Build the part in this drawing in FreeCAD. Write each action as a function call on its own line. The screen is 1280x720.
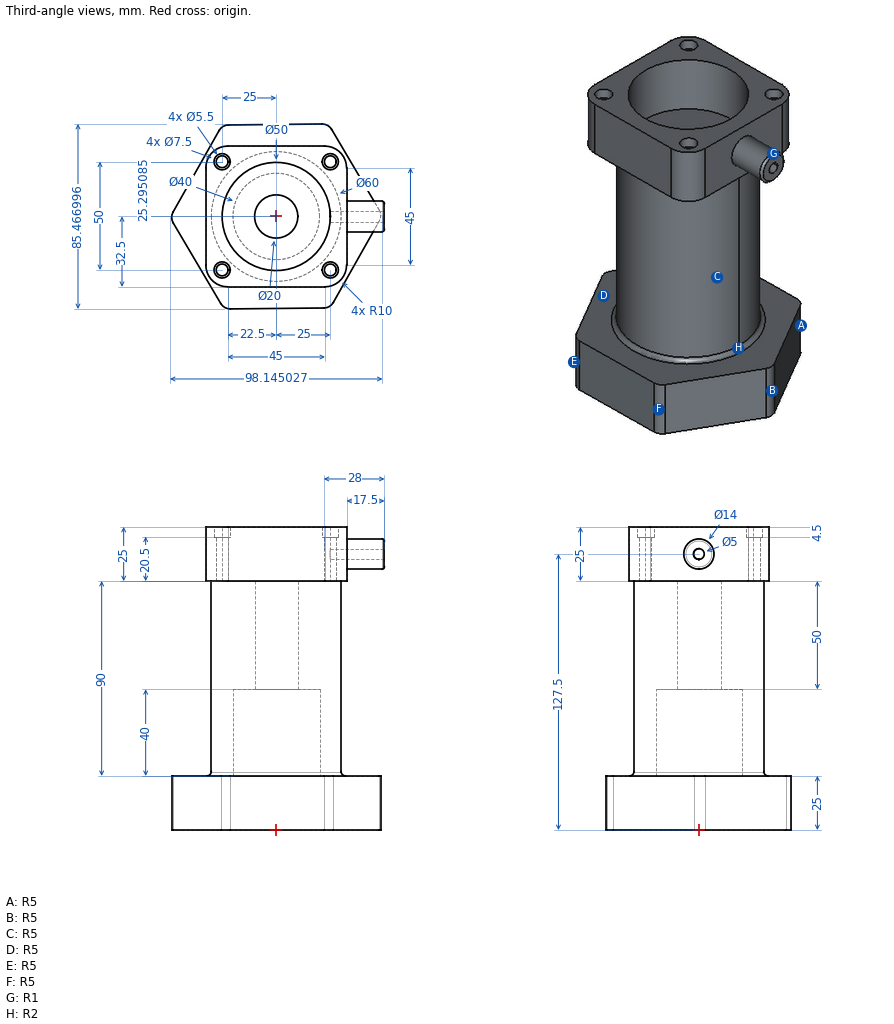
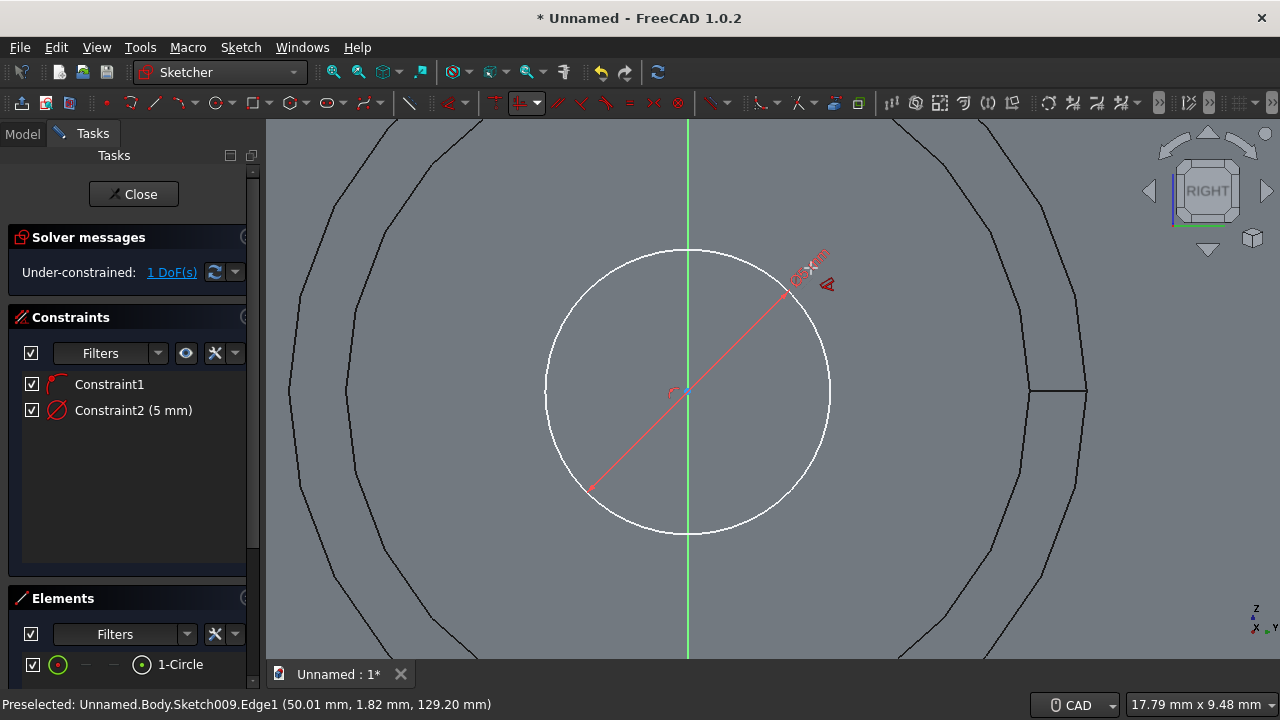
click(688, 392)
click(722, 512)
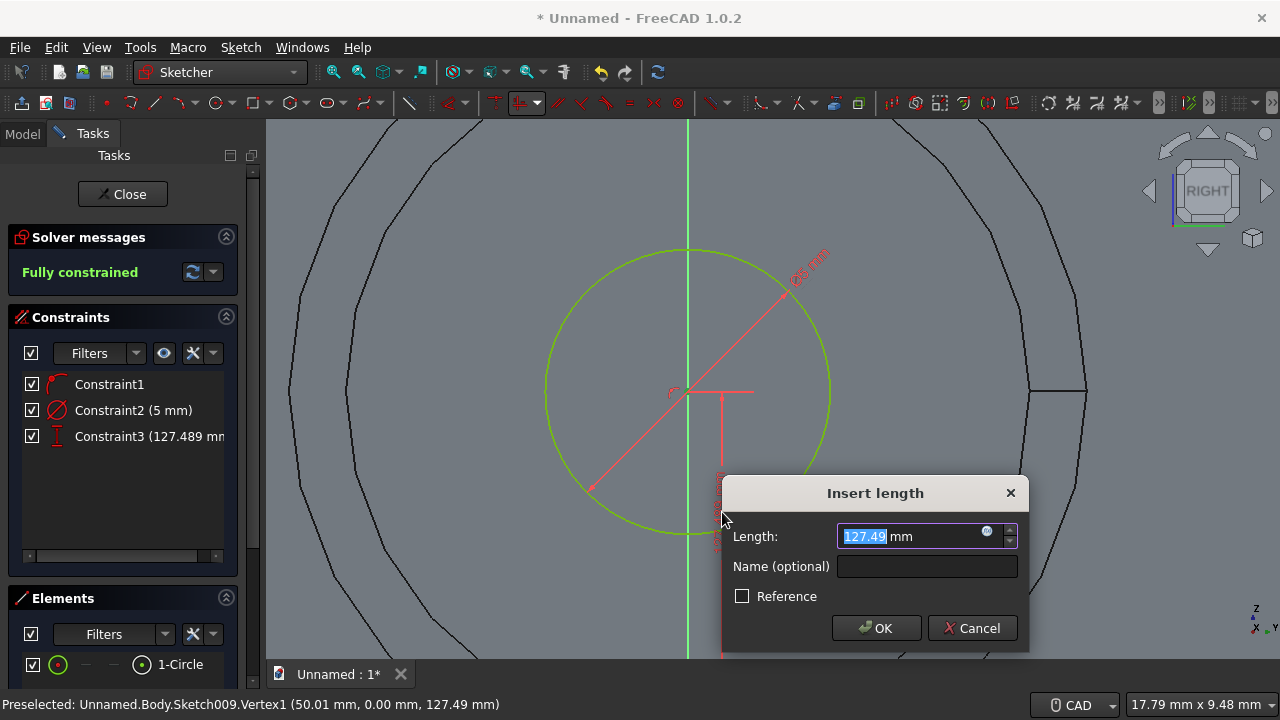
text(127.5)
key(Return)
key(Escape)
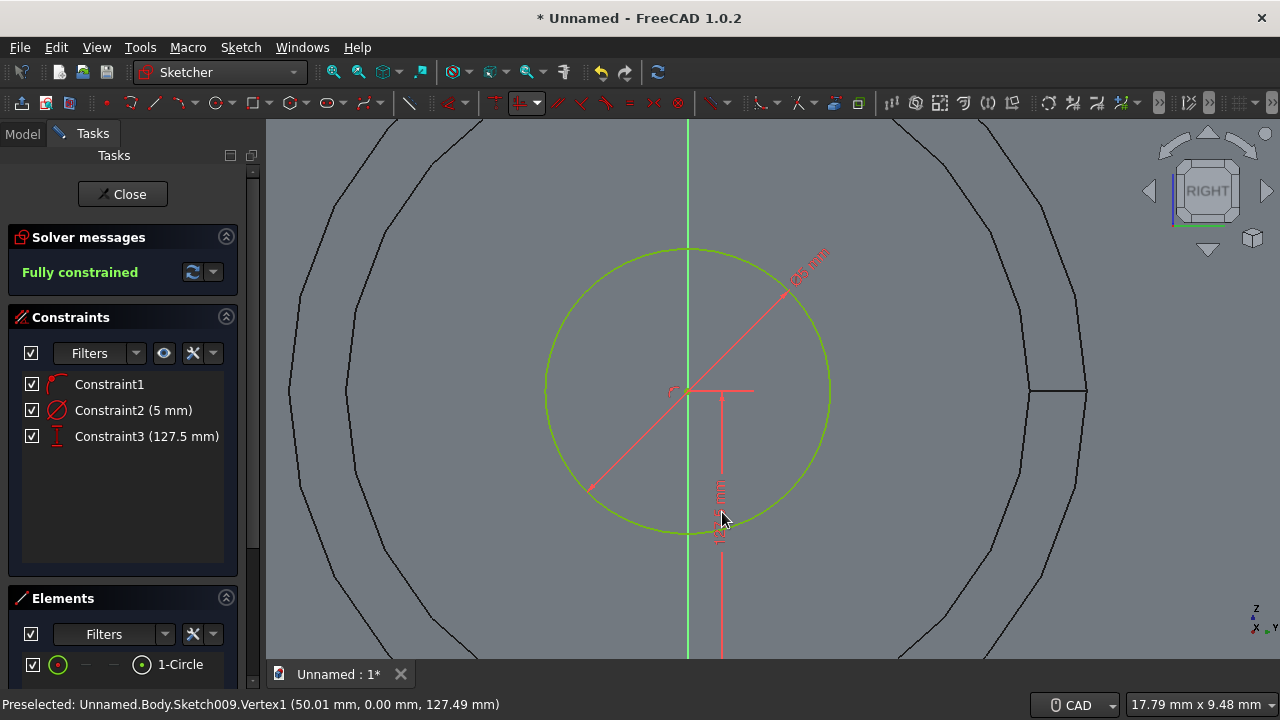
click(123, 194)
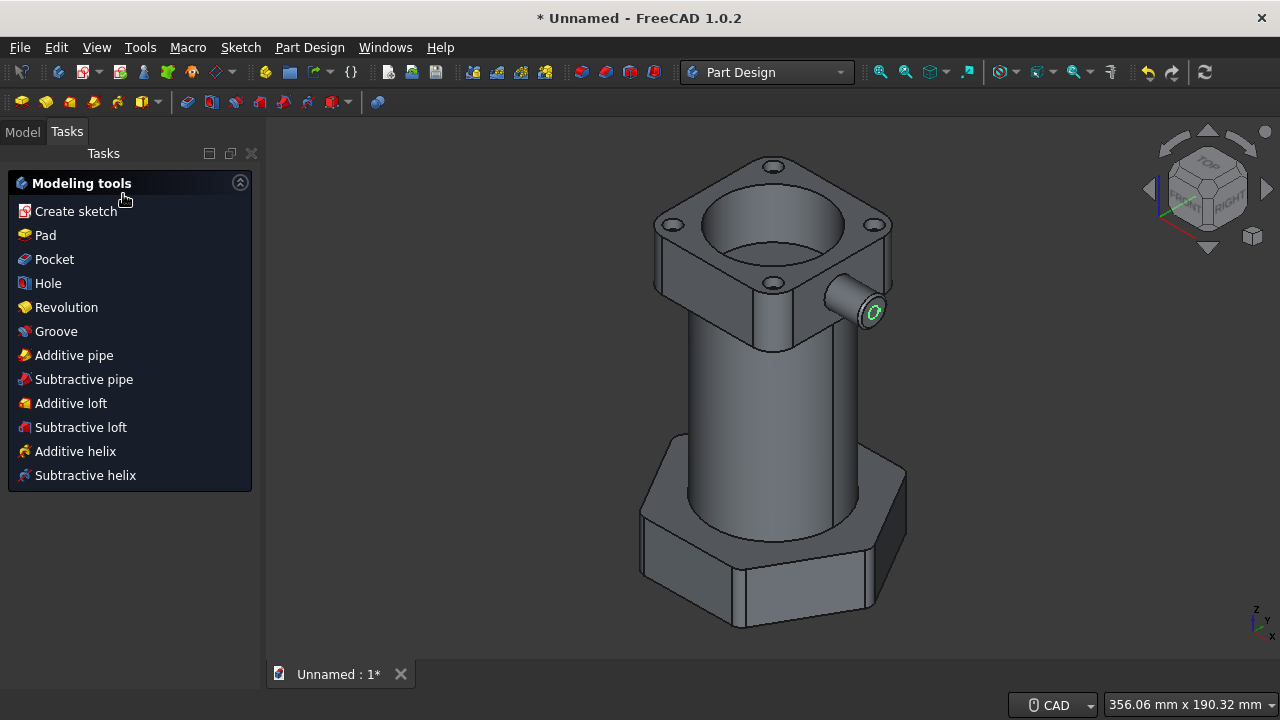
click(188, 102)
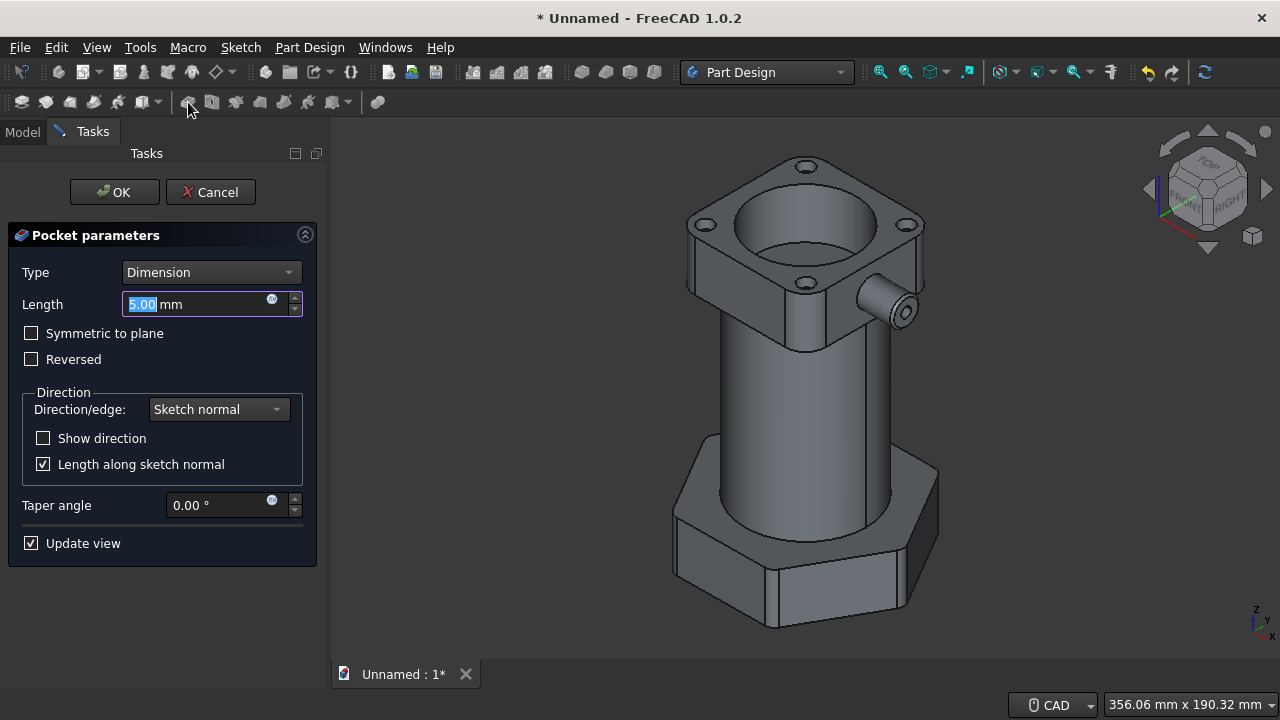
text(28)
key(Tab)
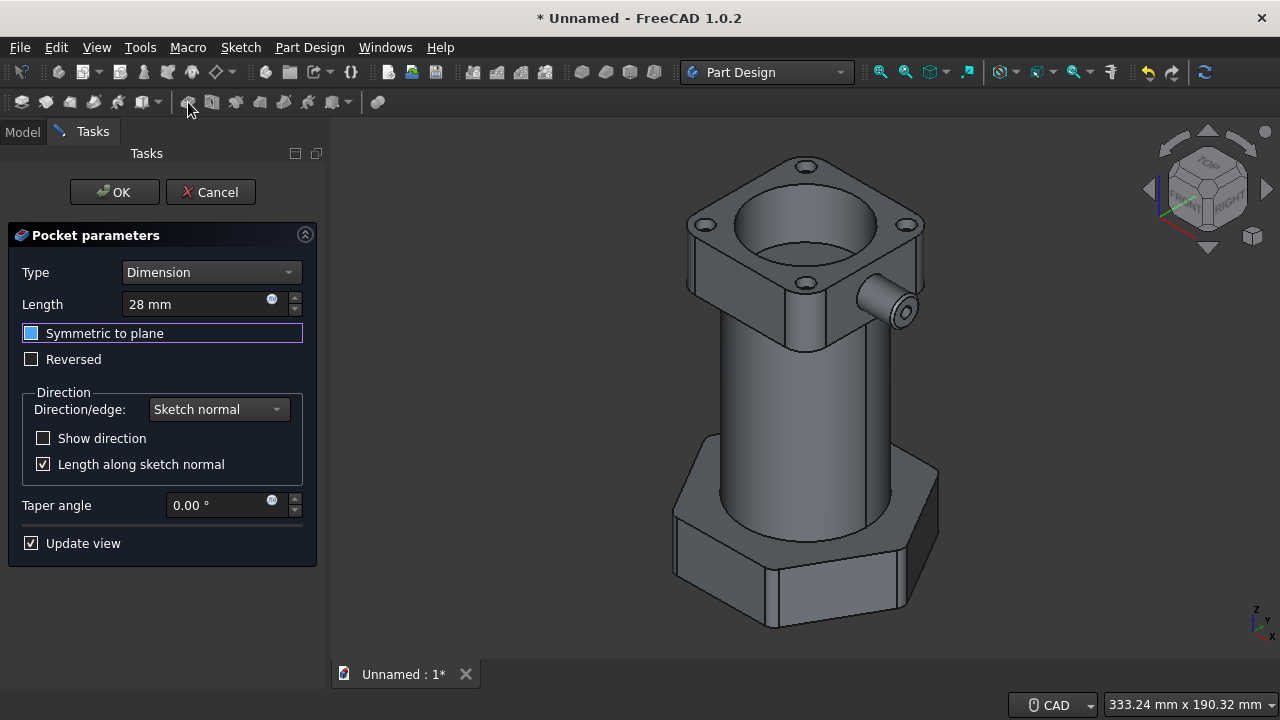
click(115, 192)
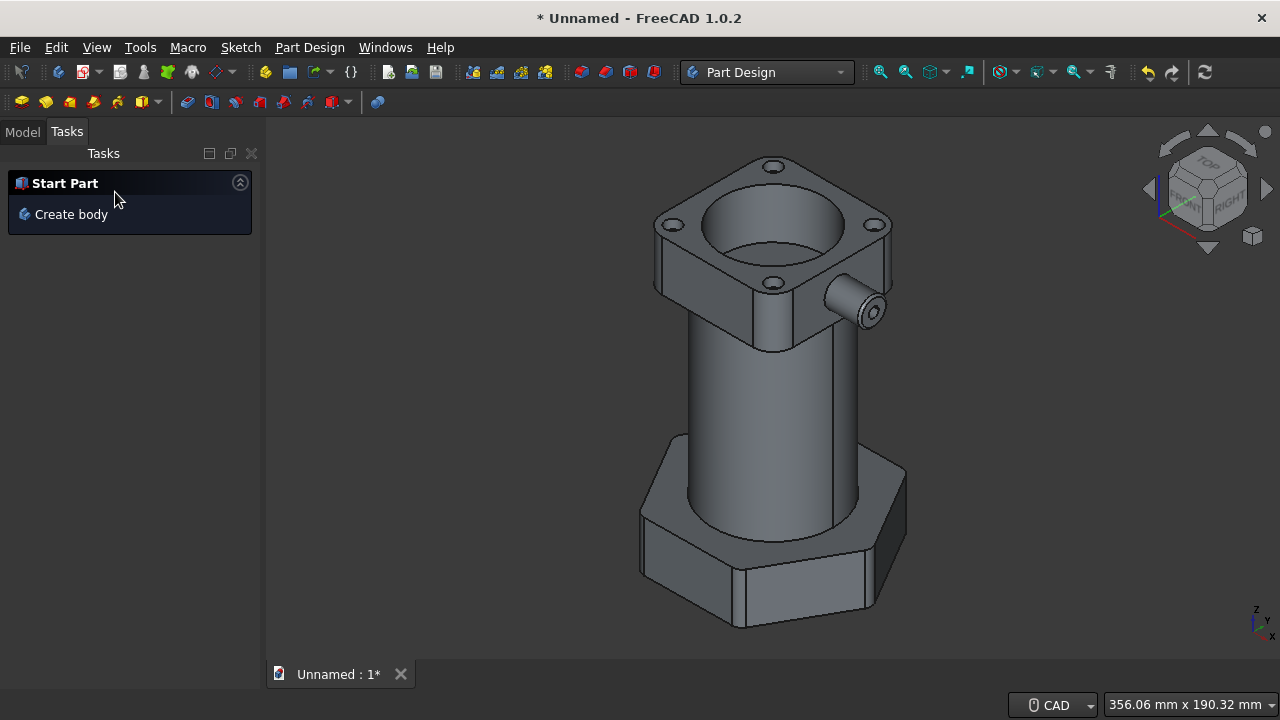
key(2)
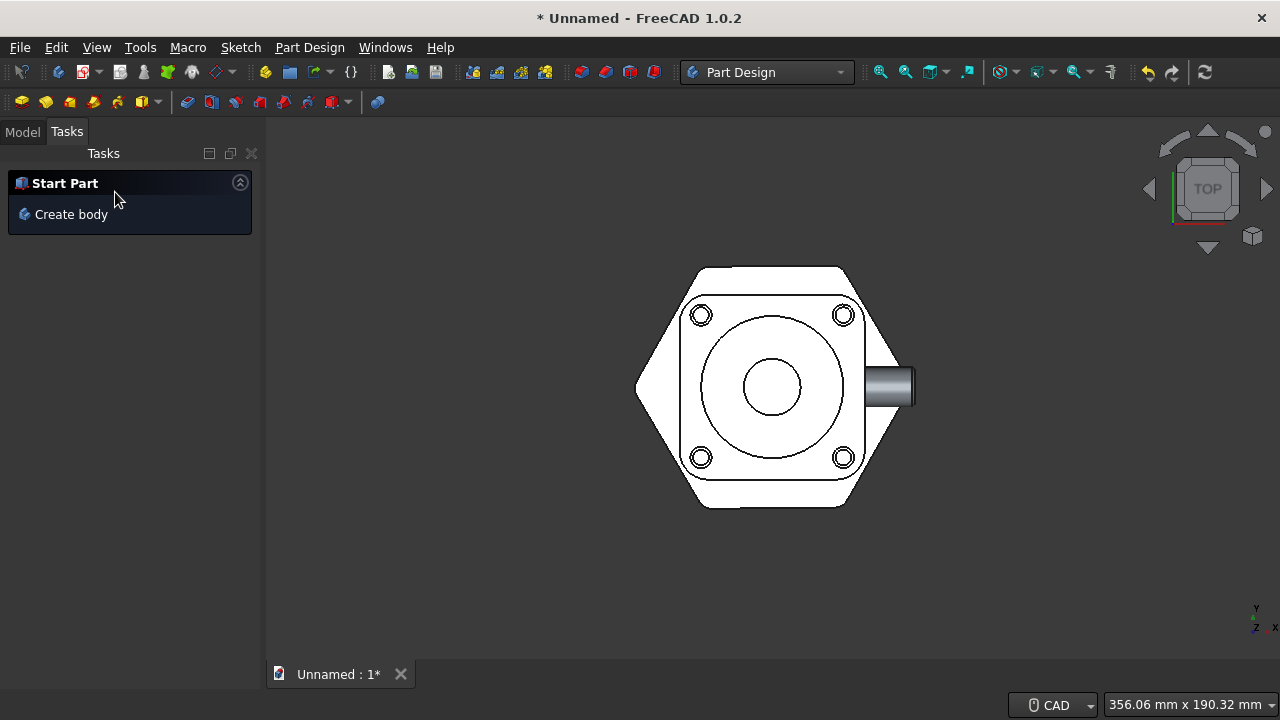
click(882, 72)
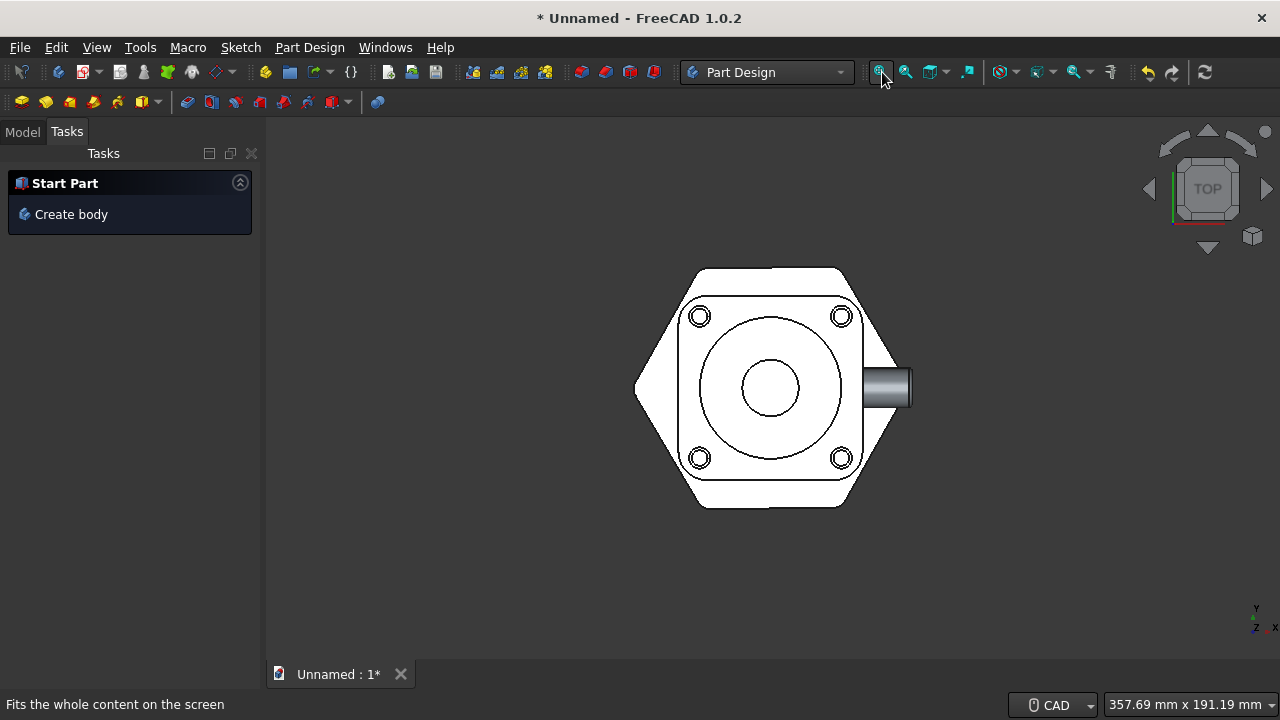
key(0)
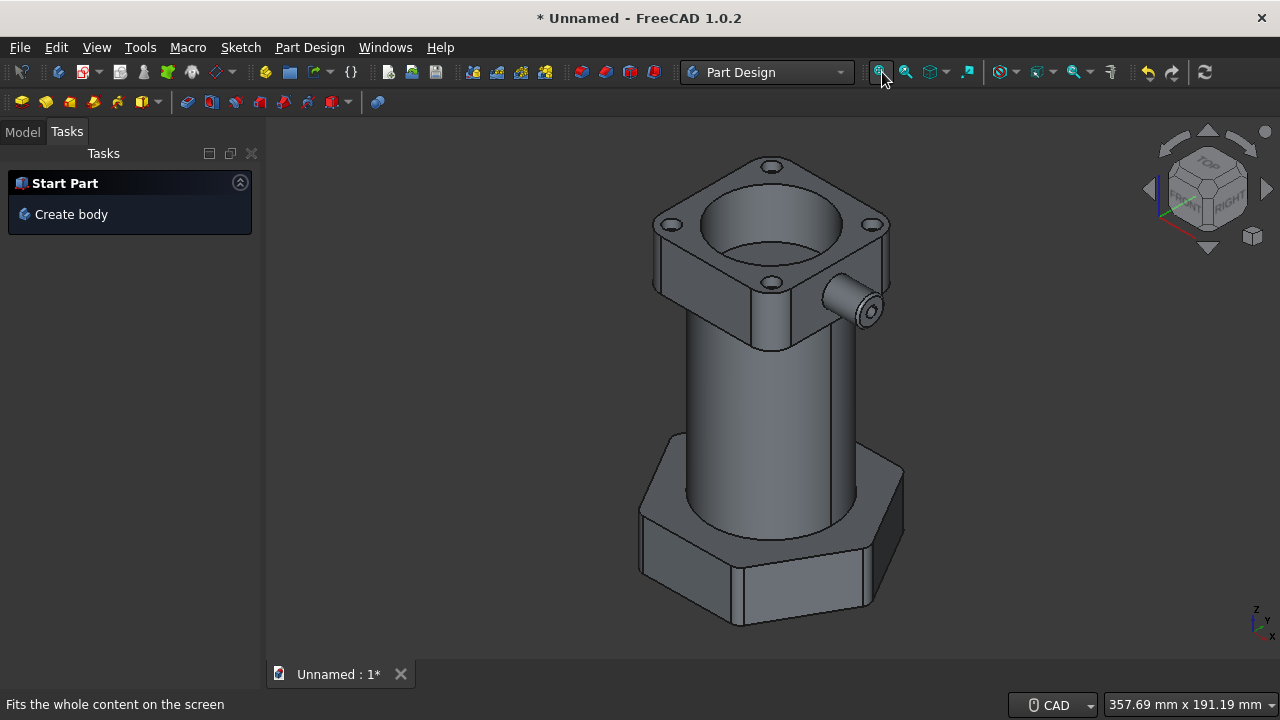
key(1)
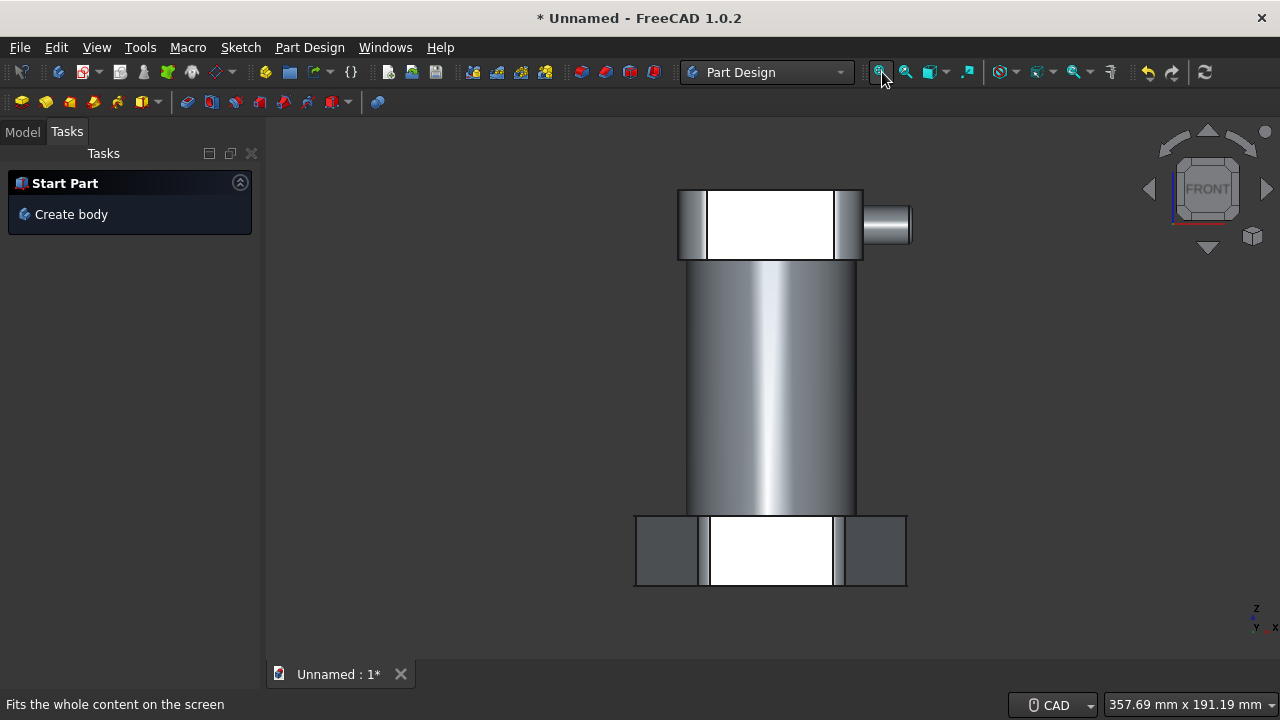
key(3)